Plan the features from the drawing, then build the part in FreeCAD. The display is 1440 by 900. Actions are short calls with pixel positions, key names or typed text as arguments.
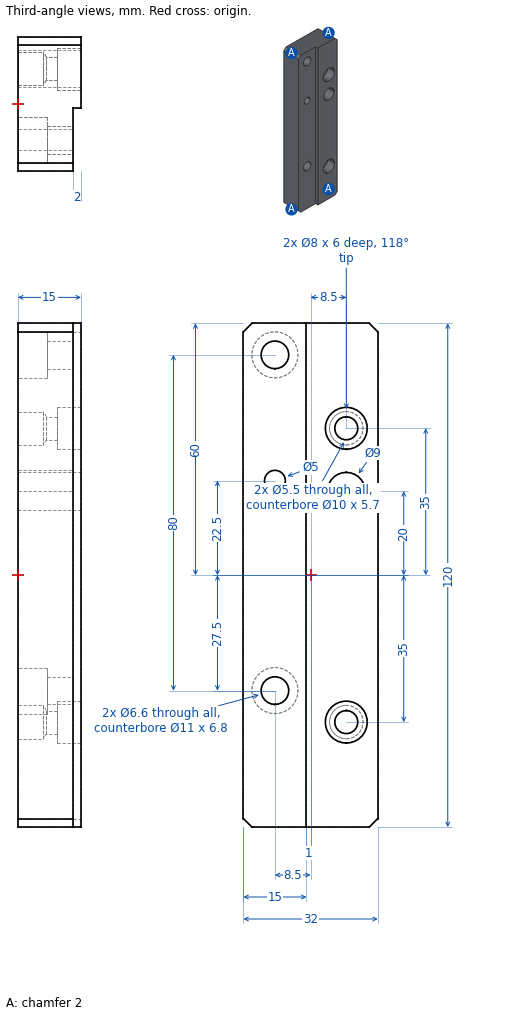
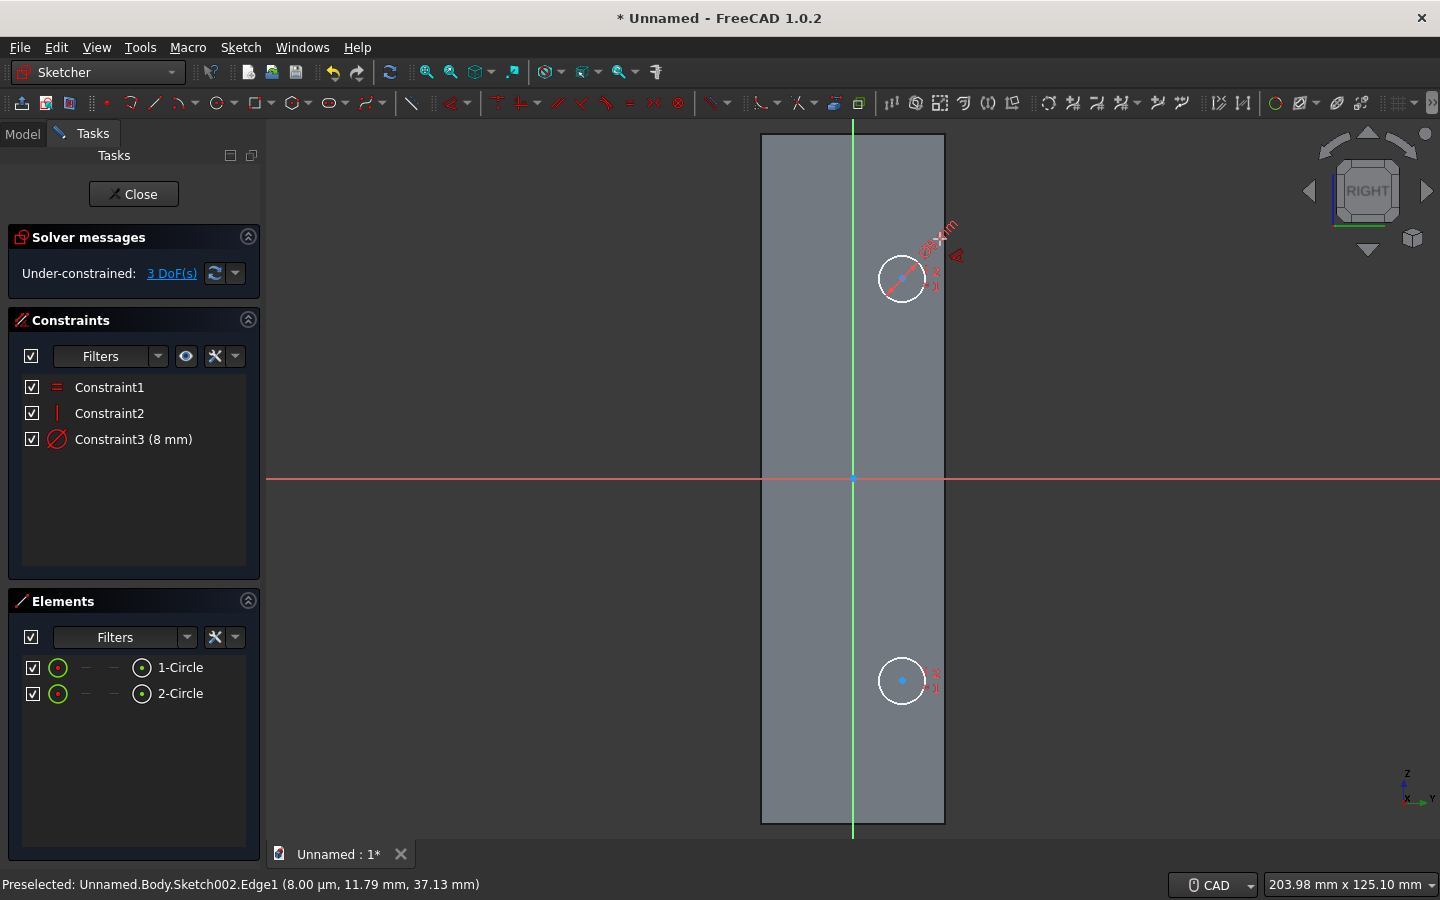
click(902, 279)
click(819, 379)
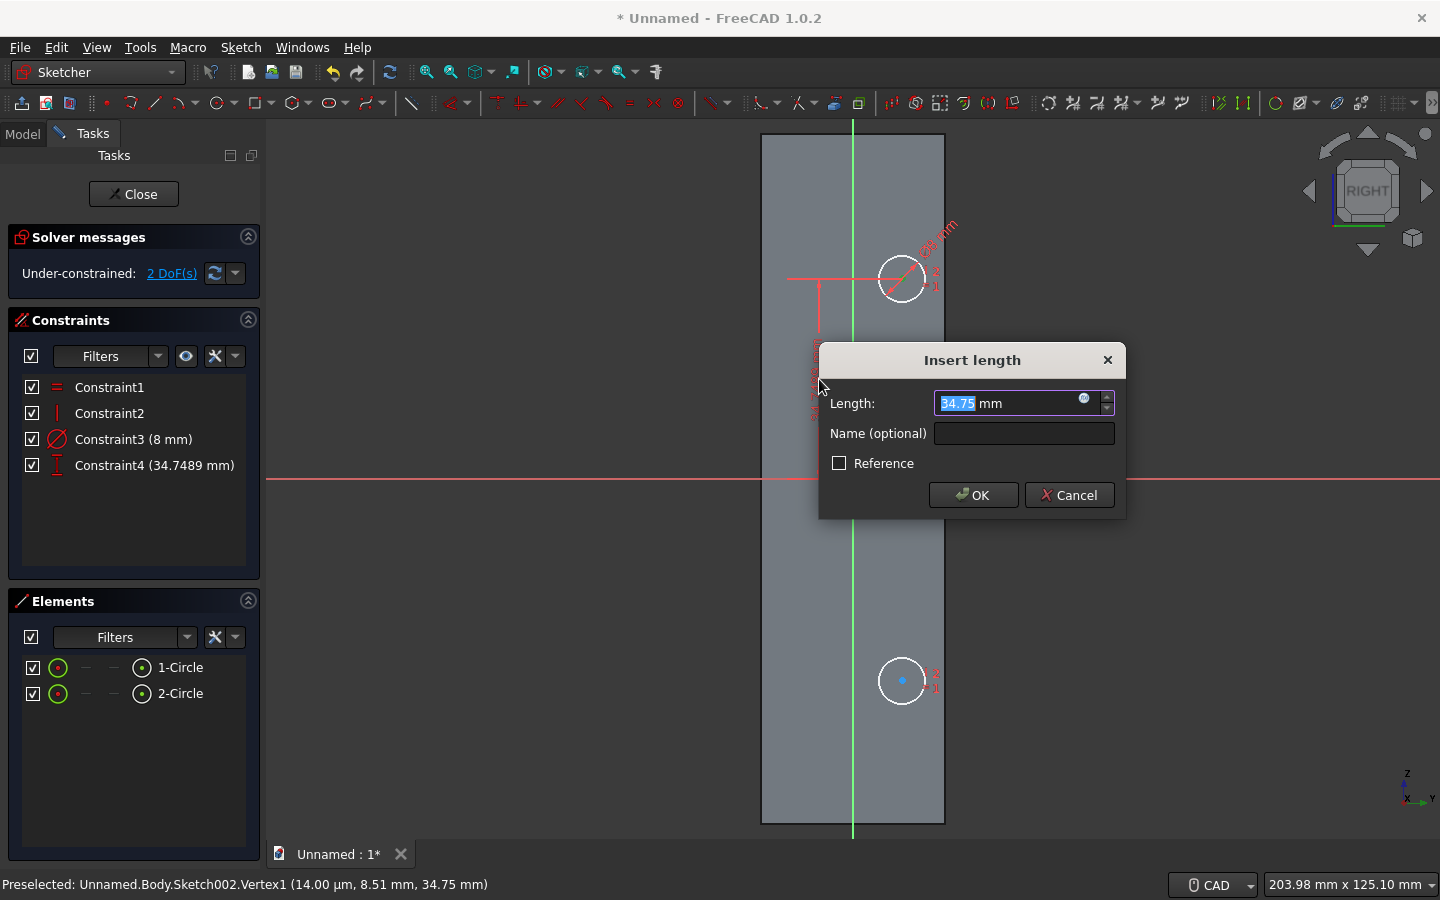
text(35)
key(Return)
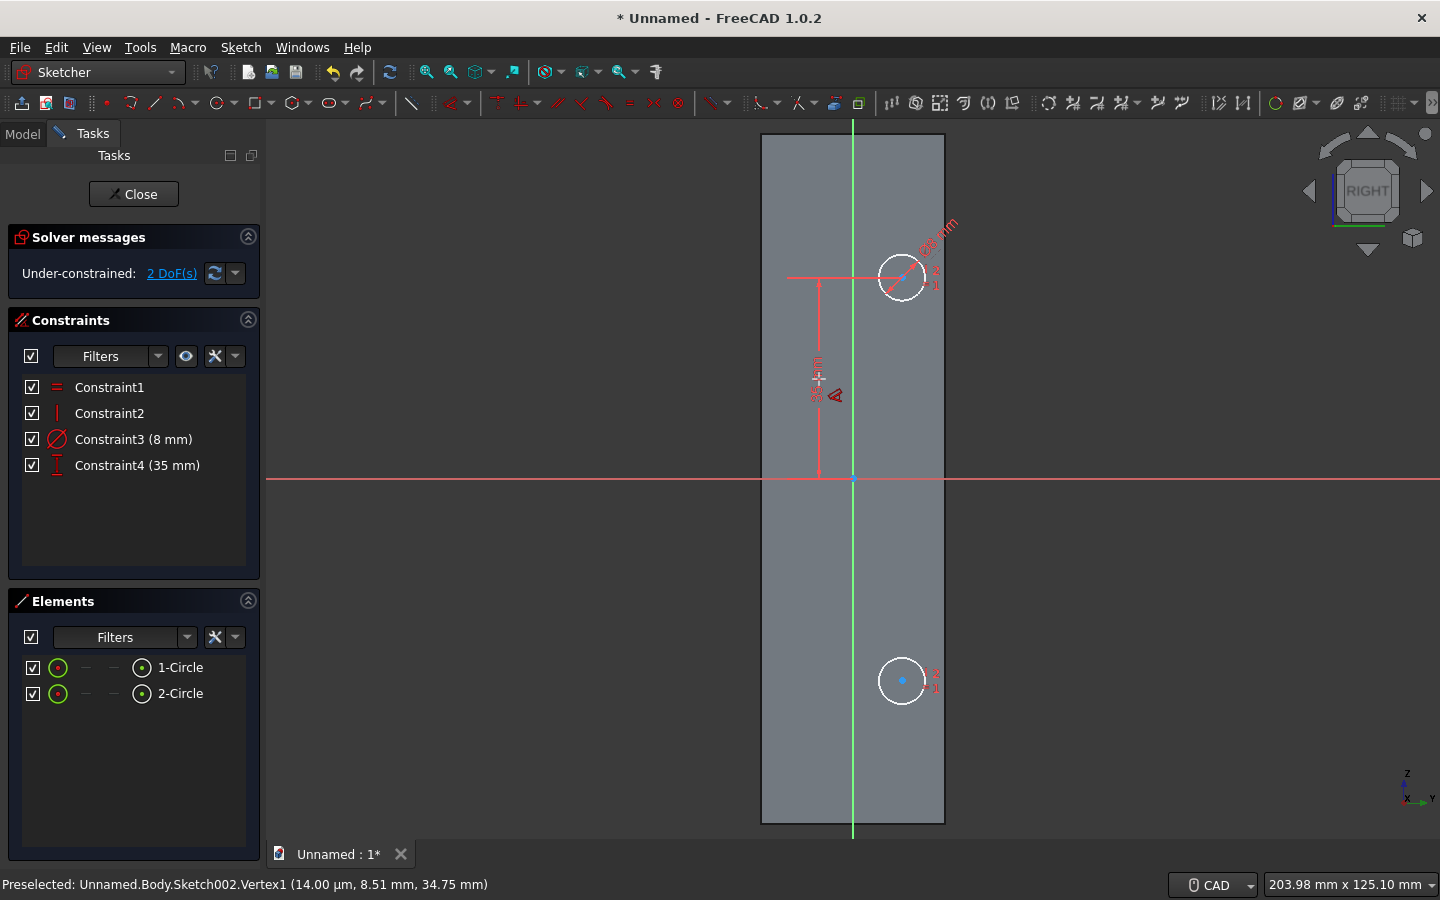
click(902, 681)
click(819, 580)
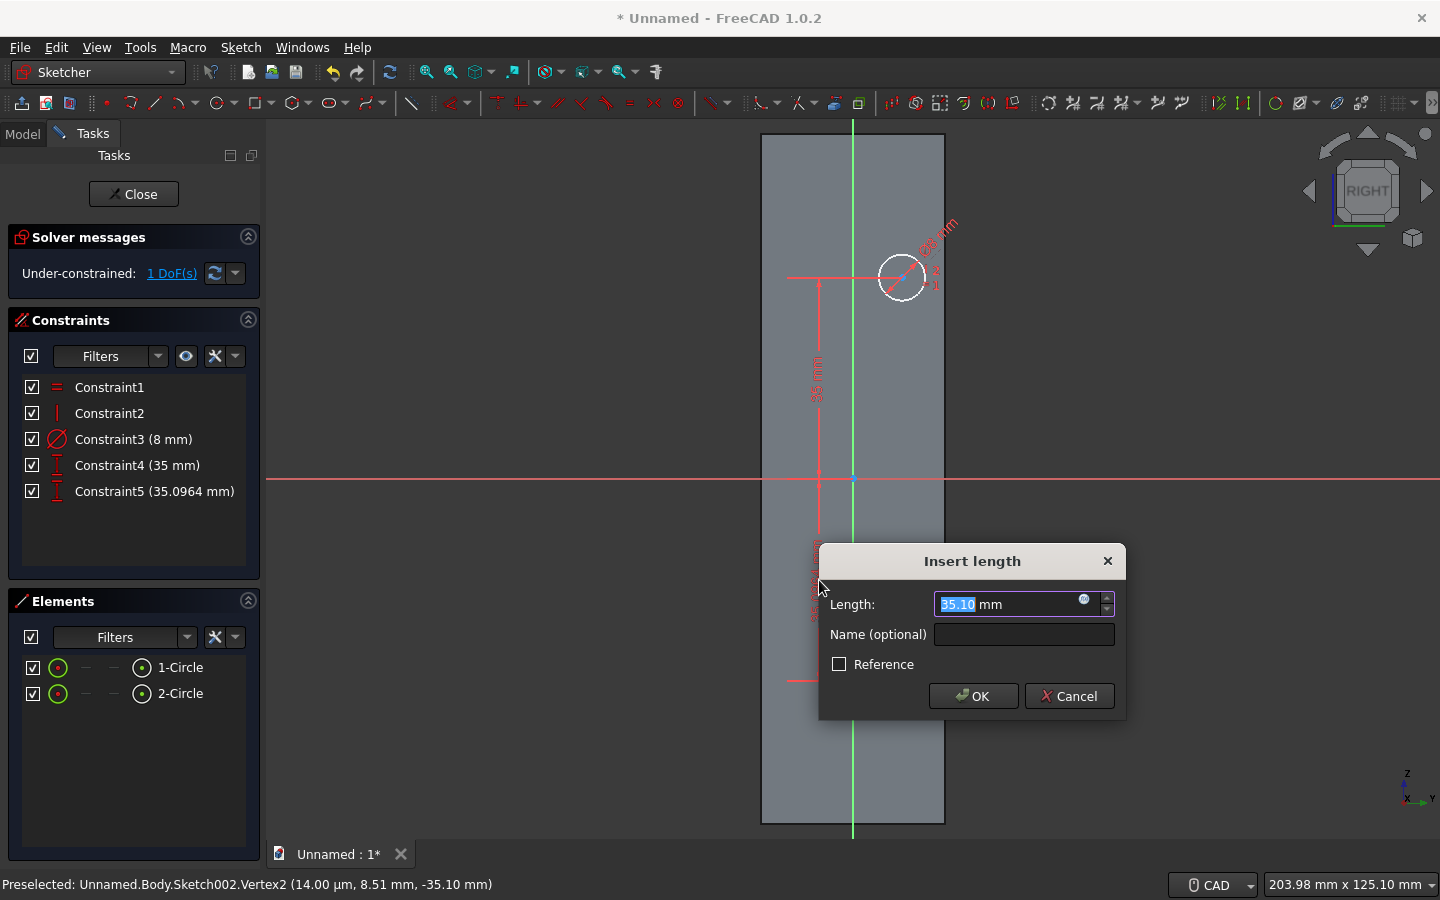
text(35)
key(Return)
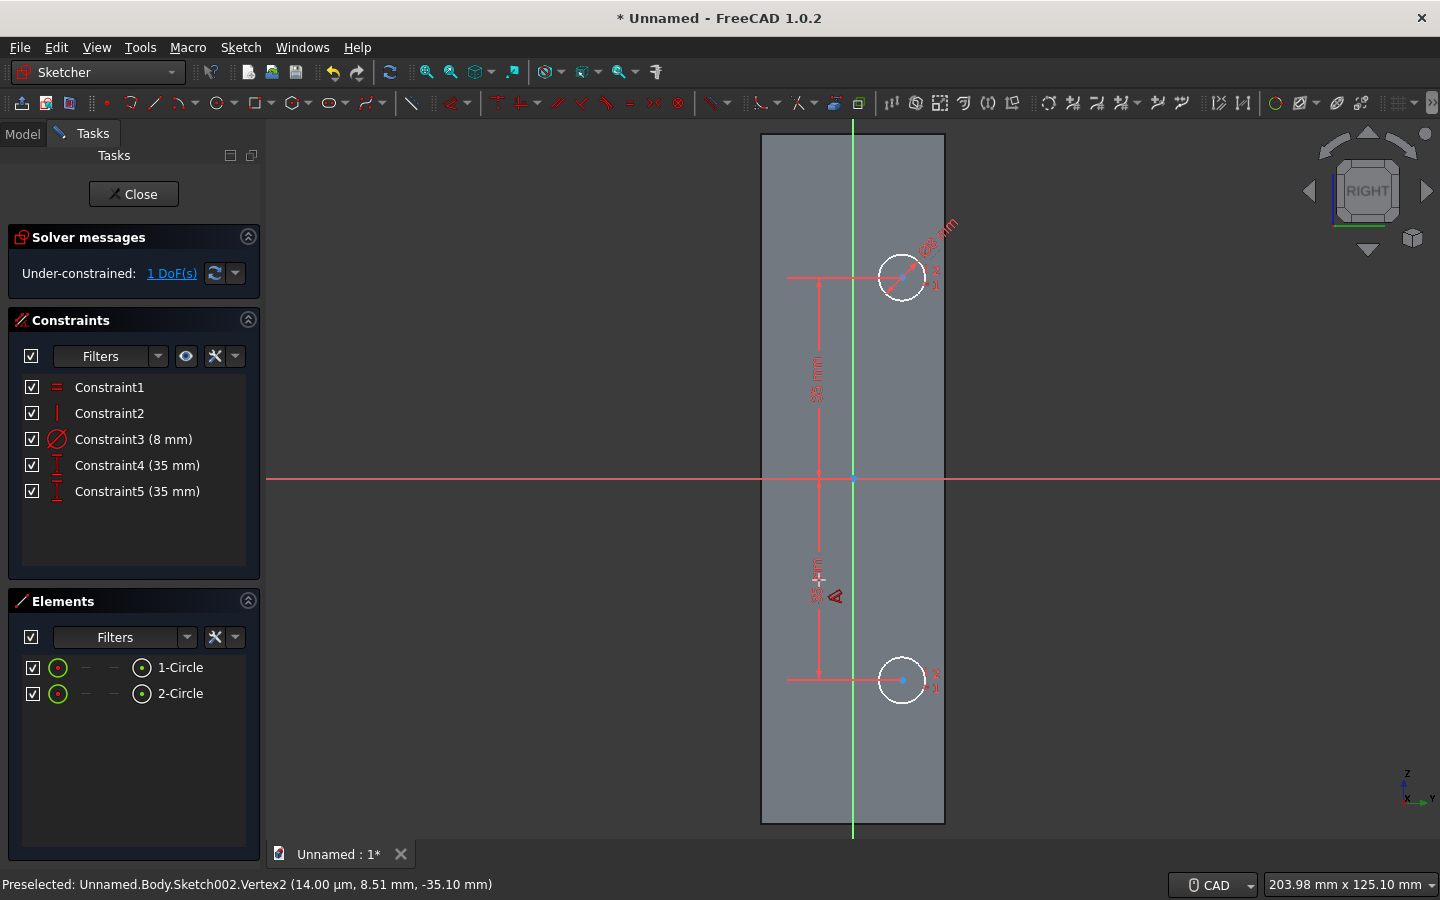
click(902, 278)
click(866, 244)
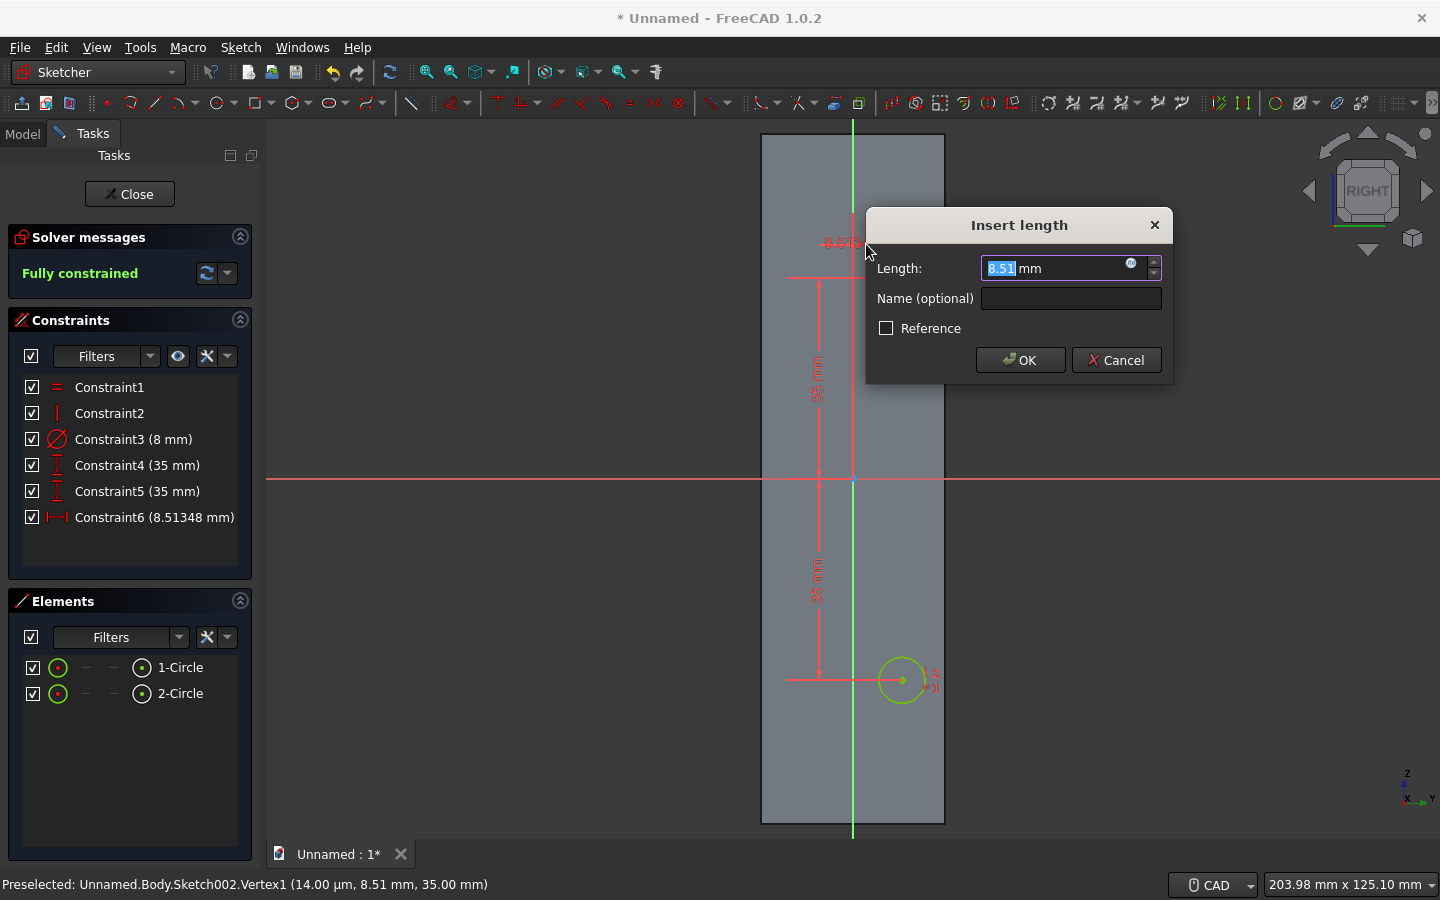
text(8.5)
key(Return)
key(Escape)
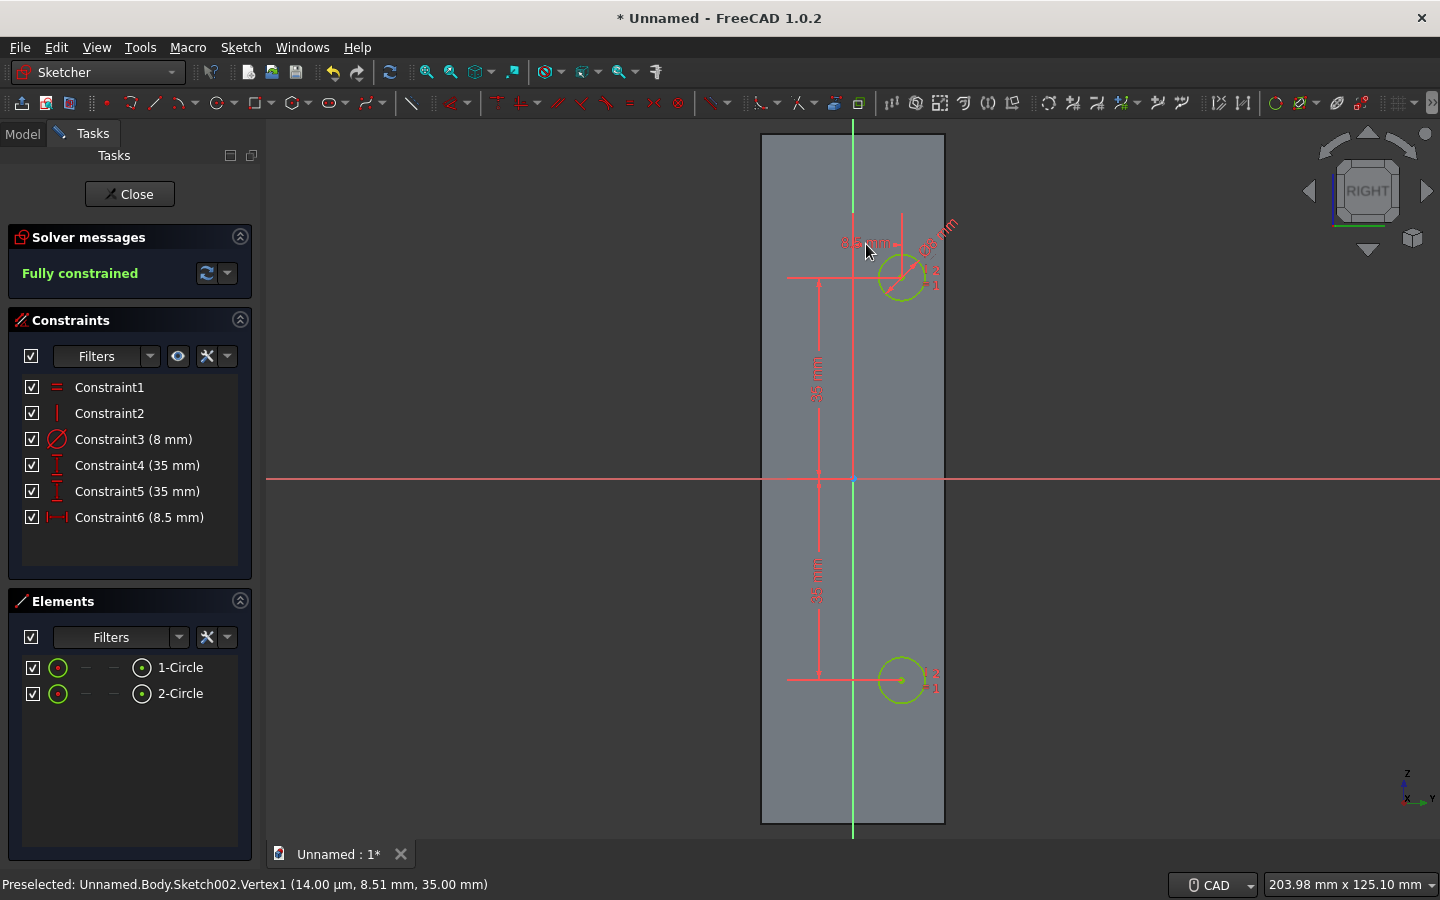
click(130, 194)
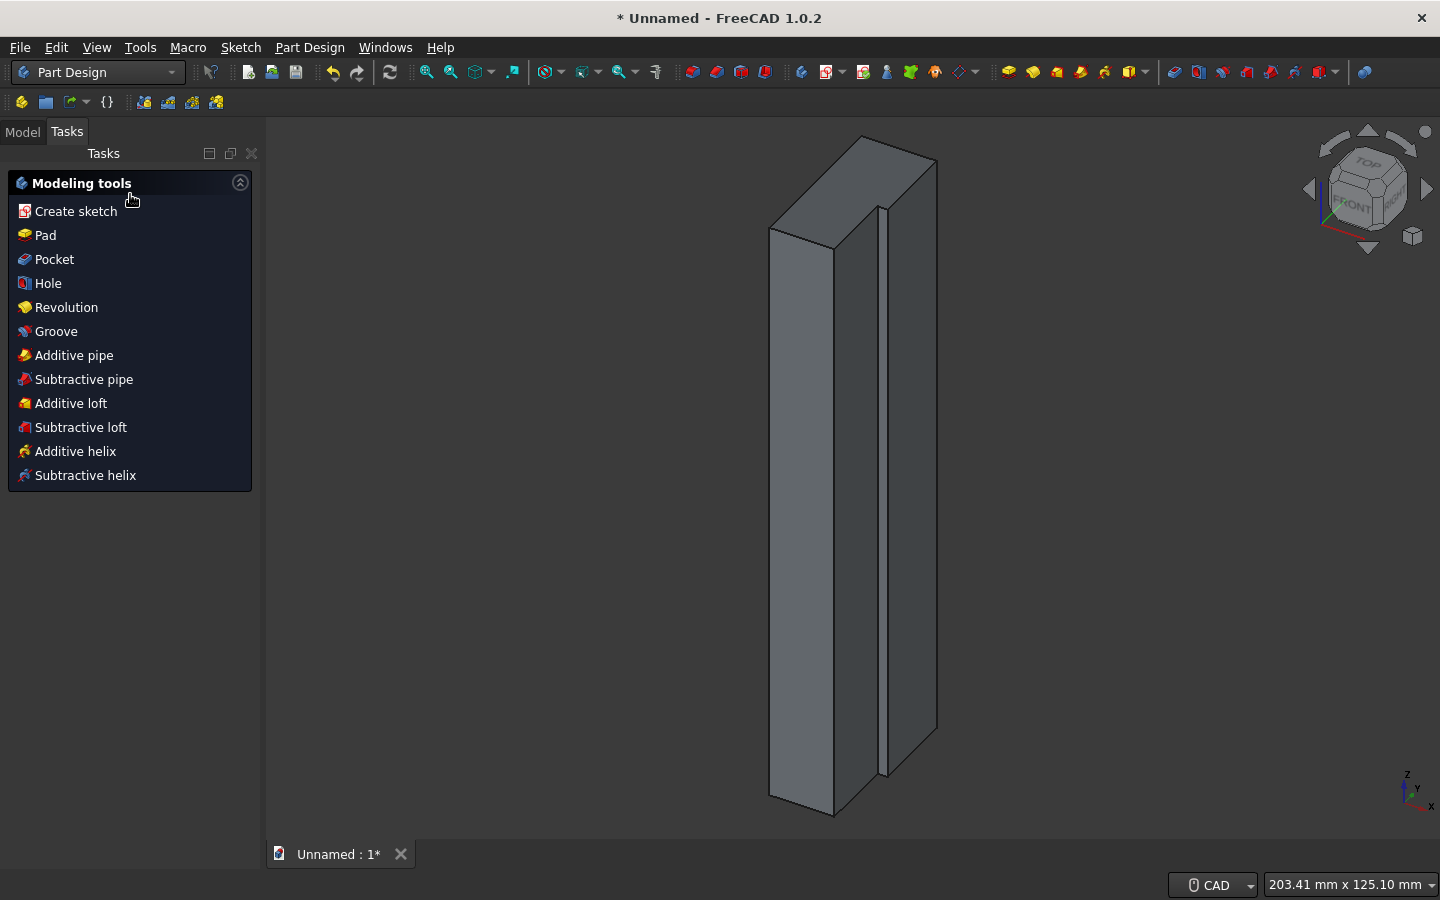
click(1200, 72)